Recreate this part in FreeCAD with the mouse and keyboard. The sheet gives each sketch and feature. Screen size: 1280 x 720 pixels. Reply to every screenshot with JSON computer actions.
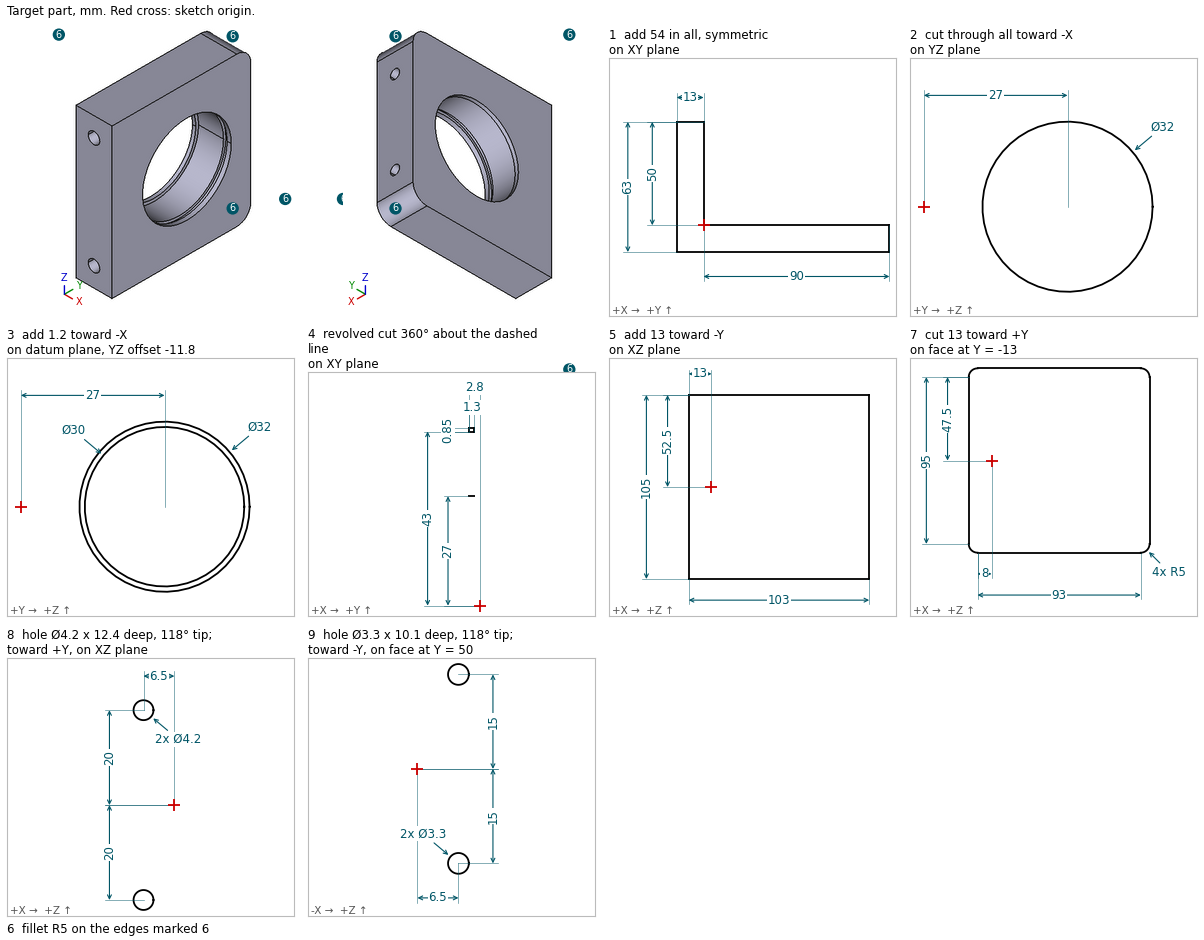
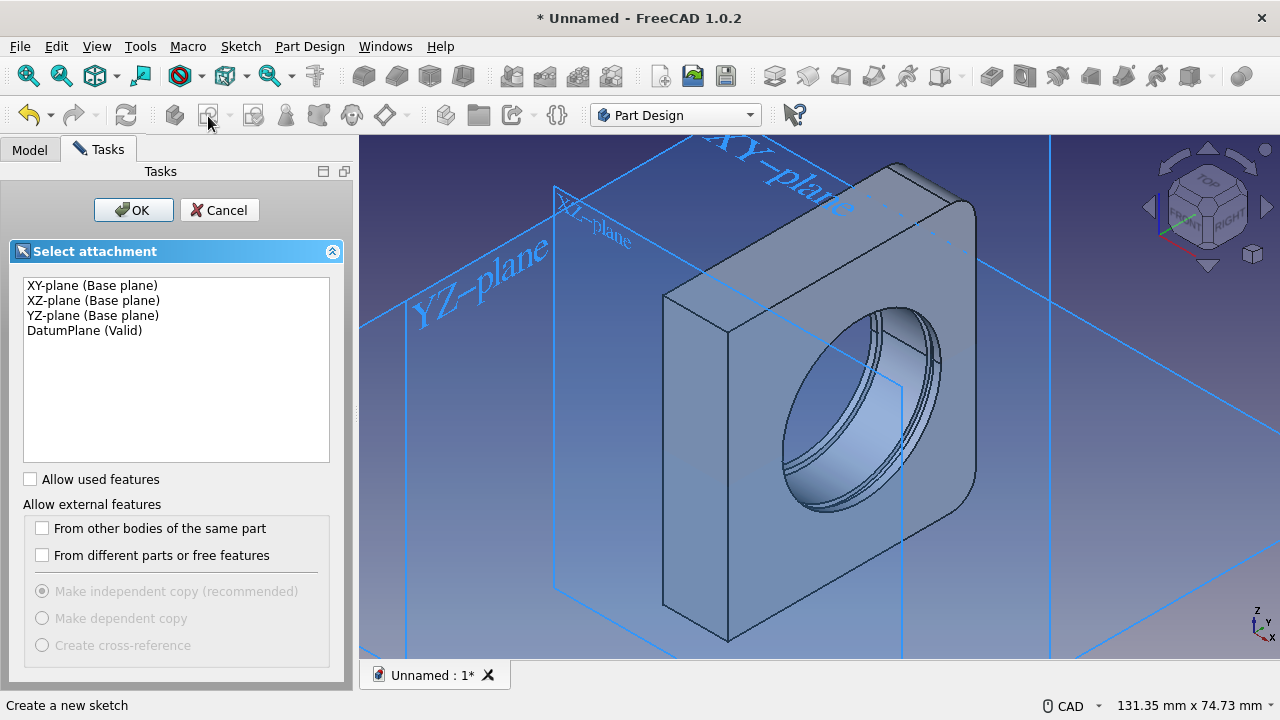
{"action": "left_click", "coordinate": [84, 300]}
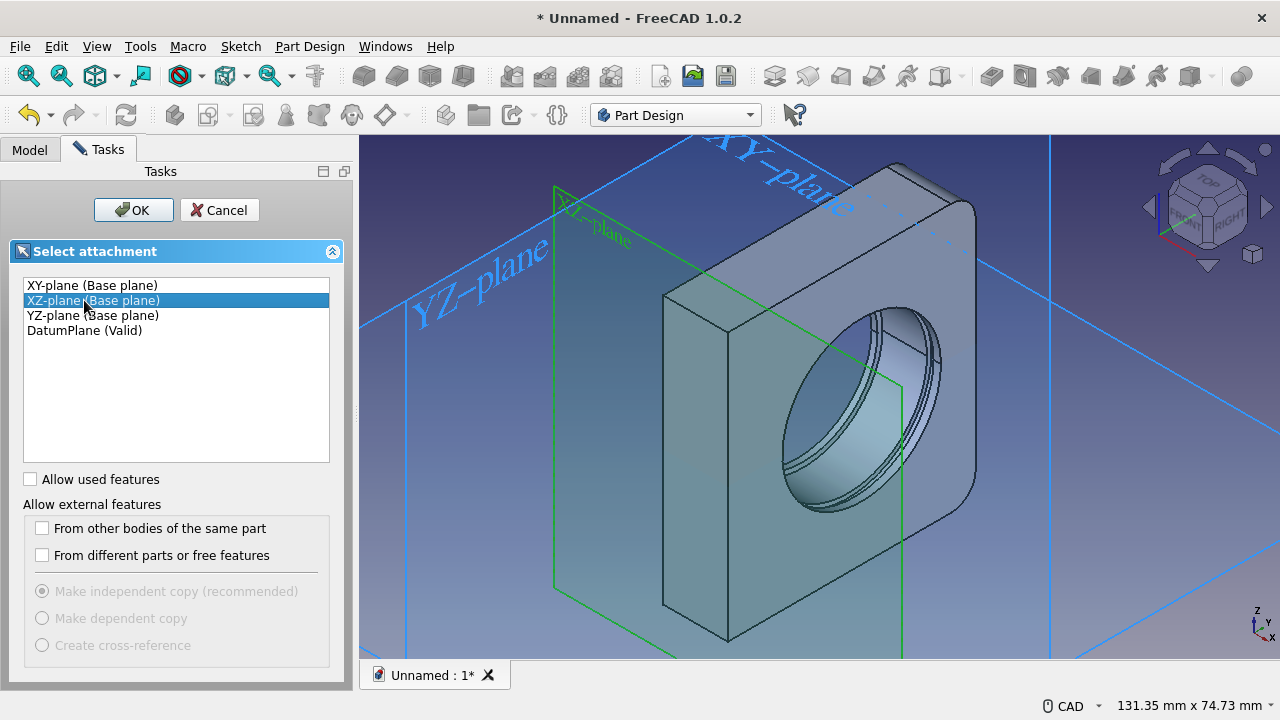
{"action": "left_click", "coordinate": [134, 210]}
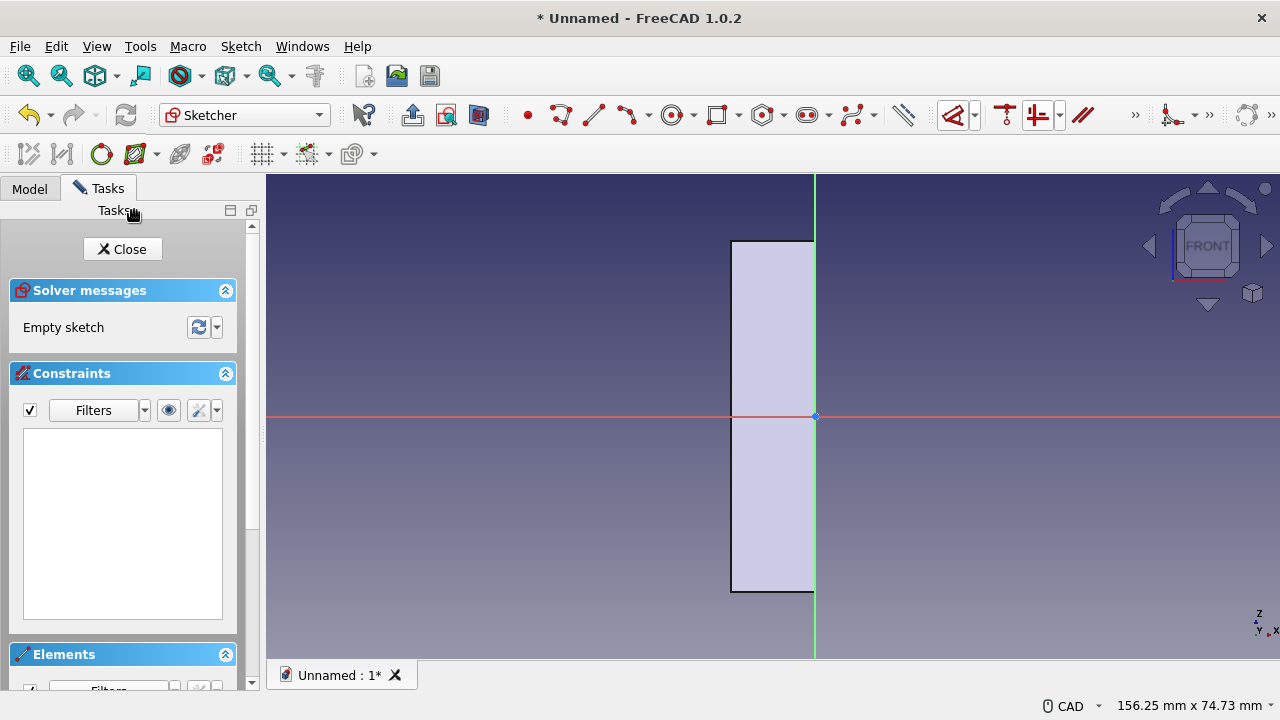
{"action": "left_click", "coordinate": [672, 116]}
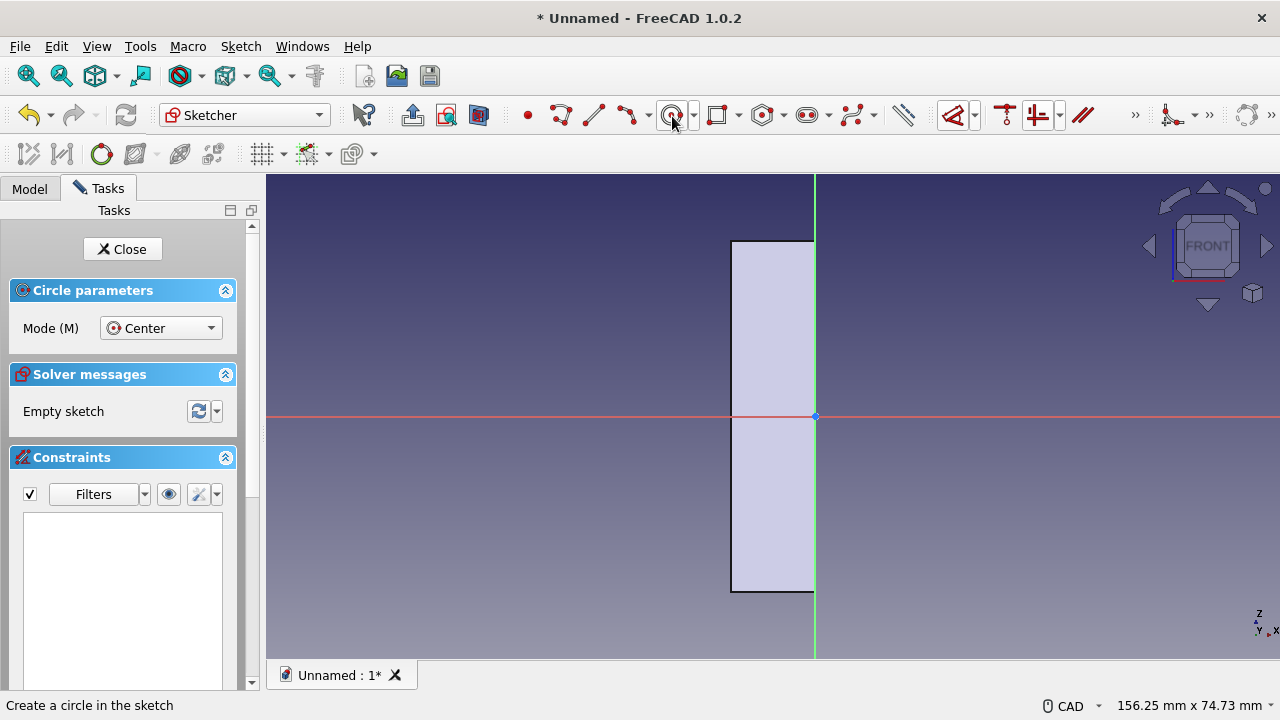
{"action": "scroll", "coordinate": [773, 287], "scroll_direction": "up", "scroll_amount": 3}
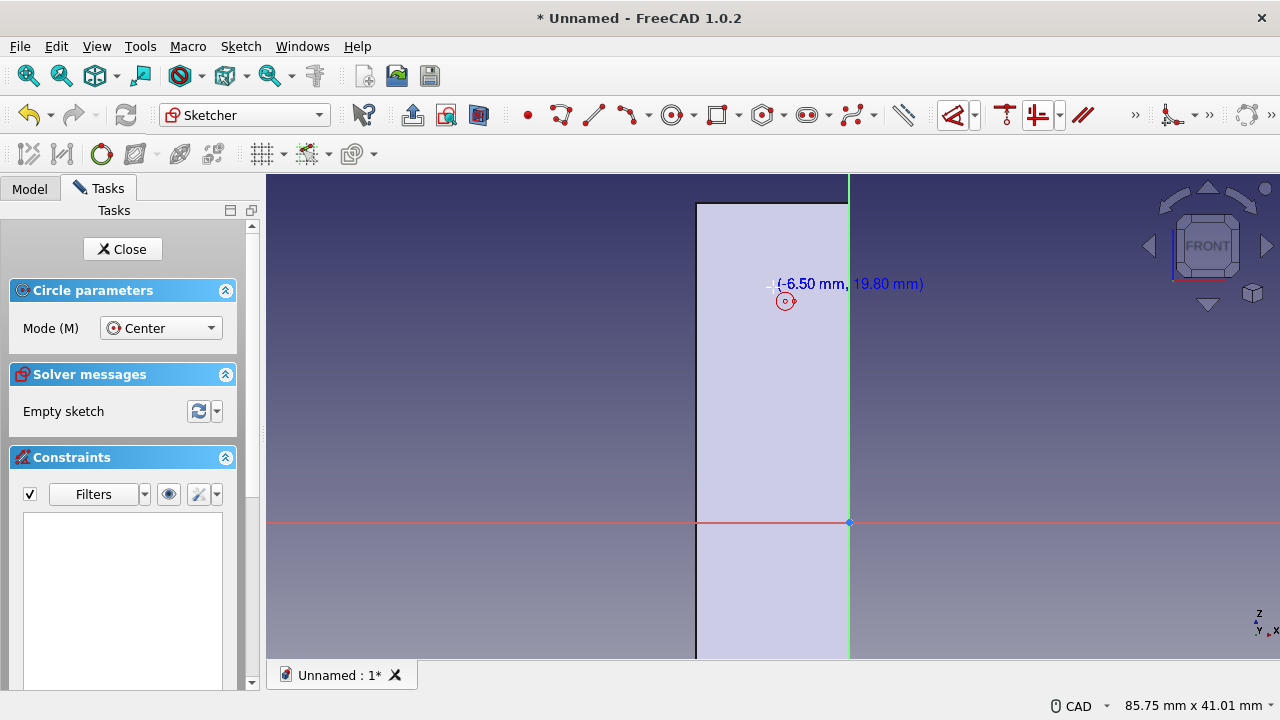
{"action": "left_click", "coordinate": [773, 286]}
{"action": "left_click", "coordinate": [790, 269]}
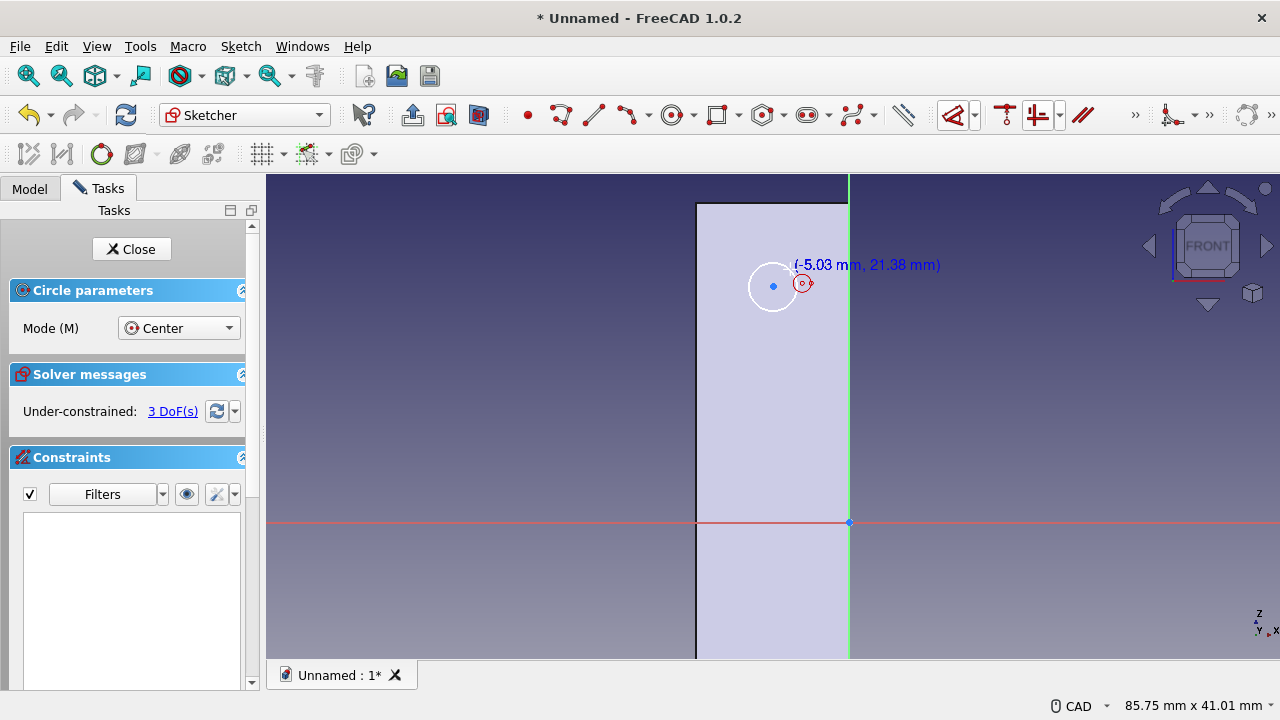
{"action": "scroll", "coordinate": [590, 287], "scroll_direction": "down", "scroll_amount": 3}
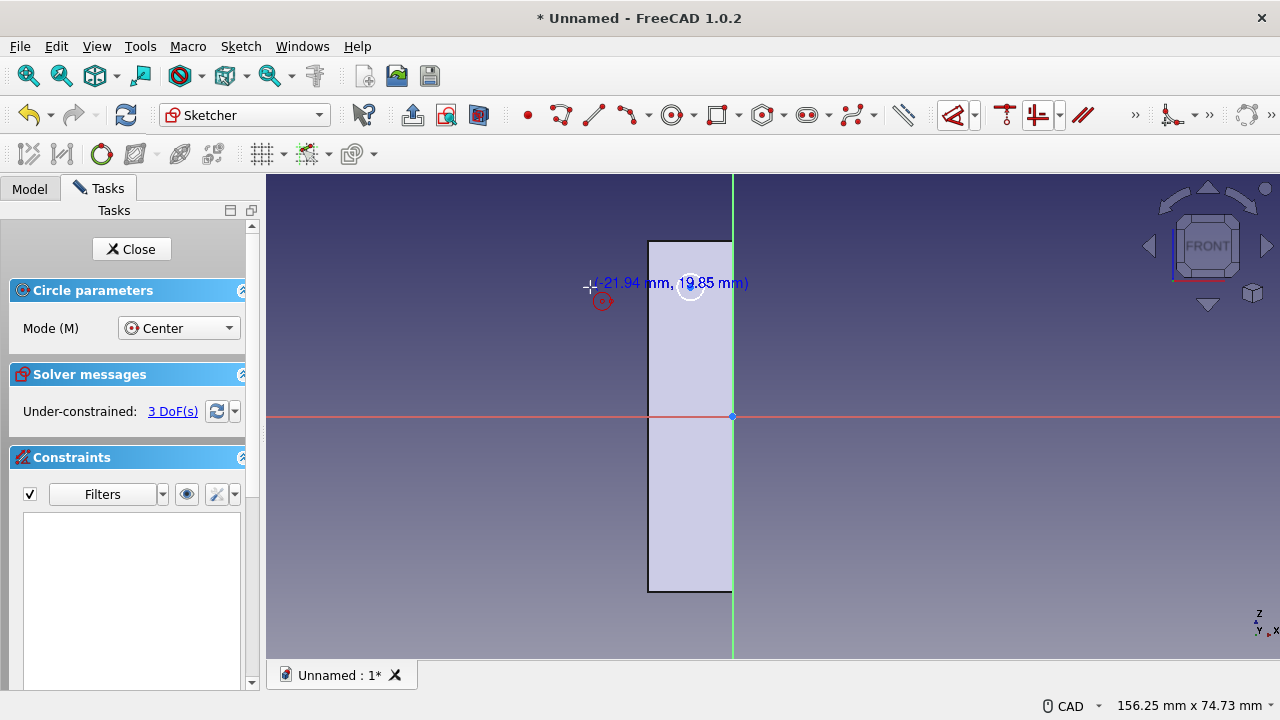
{"action": "scroll", "coordinate": [690, 546], "scroll_direction": "up", "scroll_amount": 3}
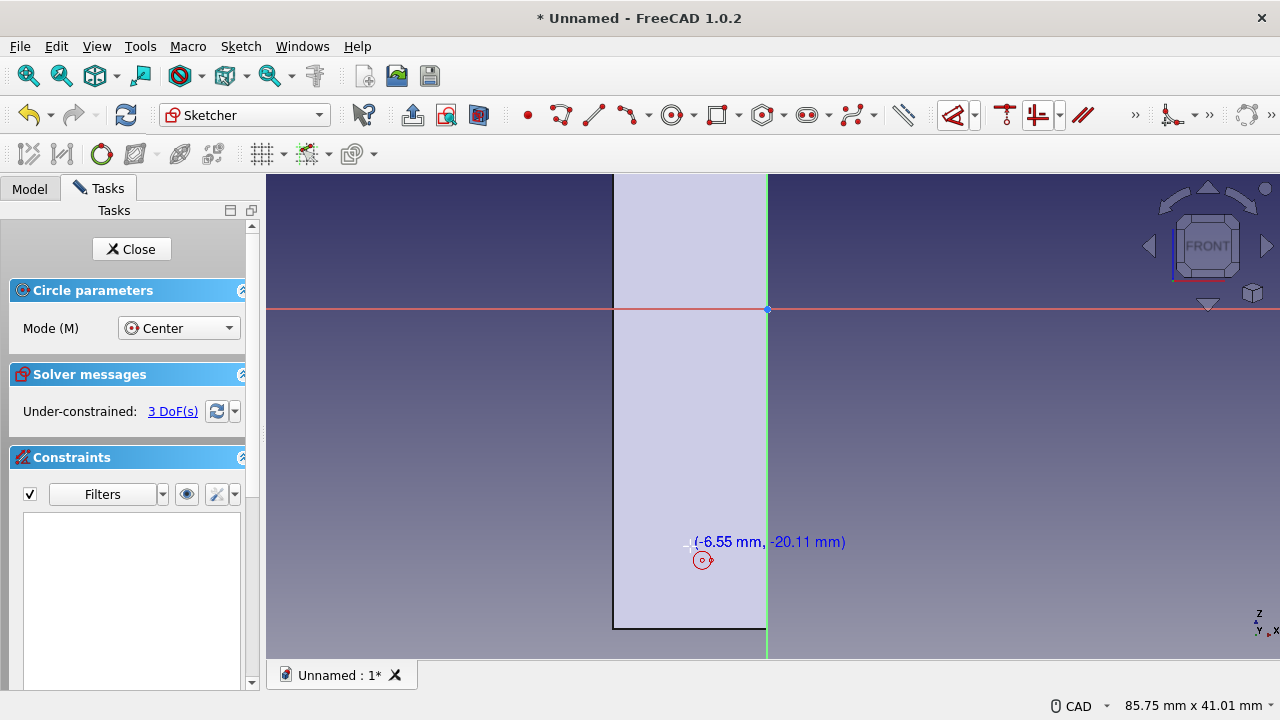
{"action": "left_click", "coordinate": [690, 546]}
{"action": "left_click", "coordinate": [708, 528]}
{"action": "key", "text": "Escape"}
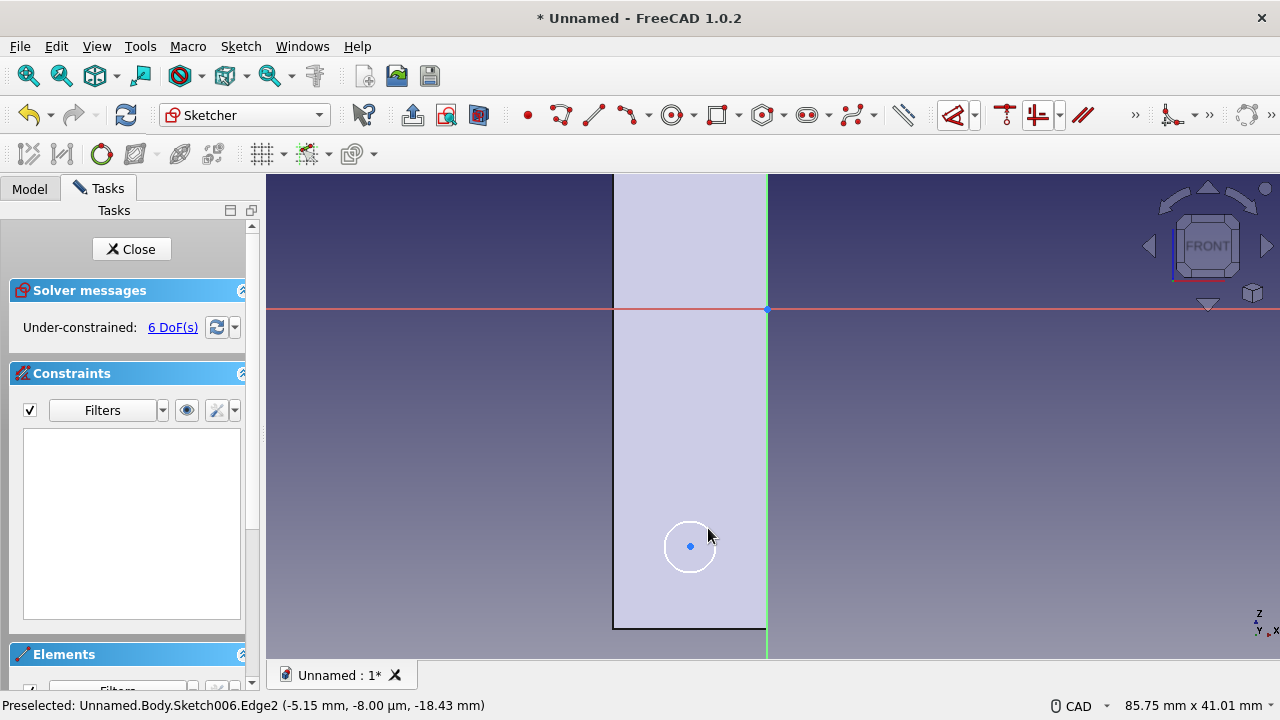
{"action": "scroll", "coordinate": [690, 547], "scroll_direction": "down", "scroll_amount": 3}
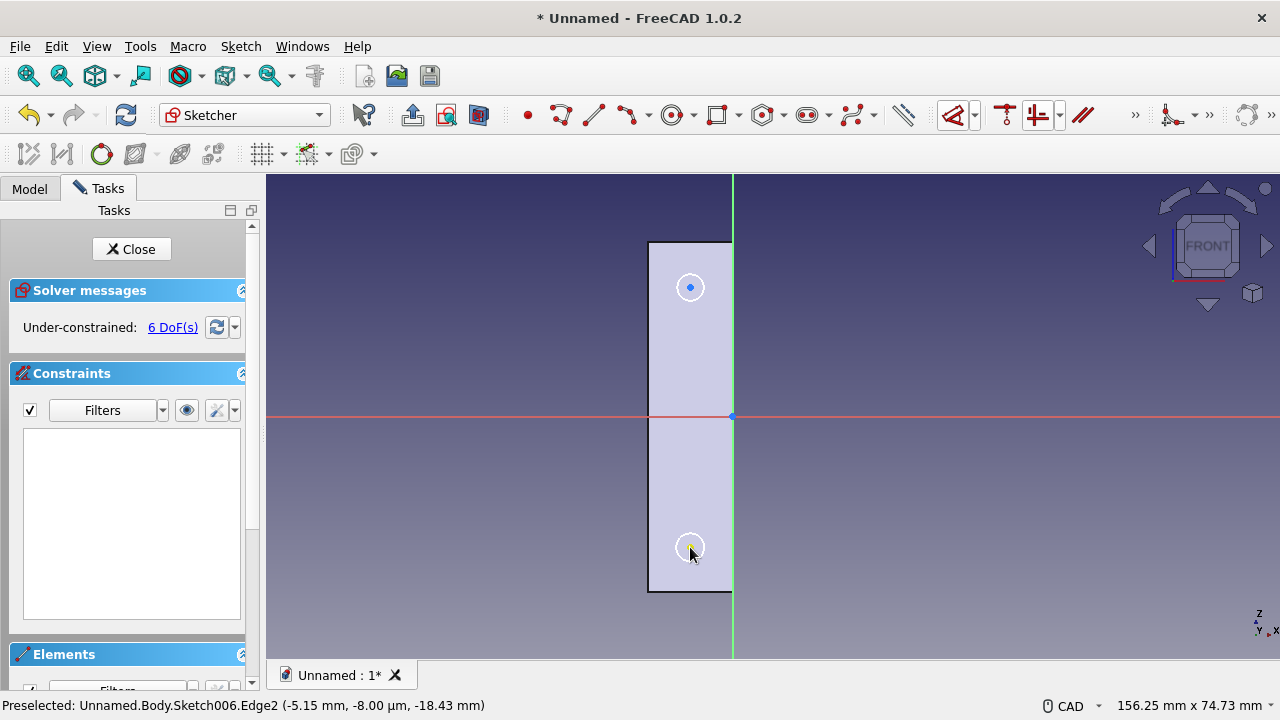
{"action": "left_click", "coordinate": [700, 278]}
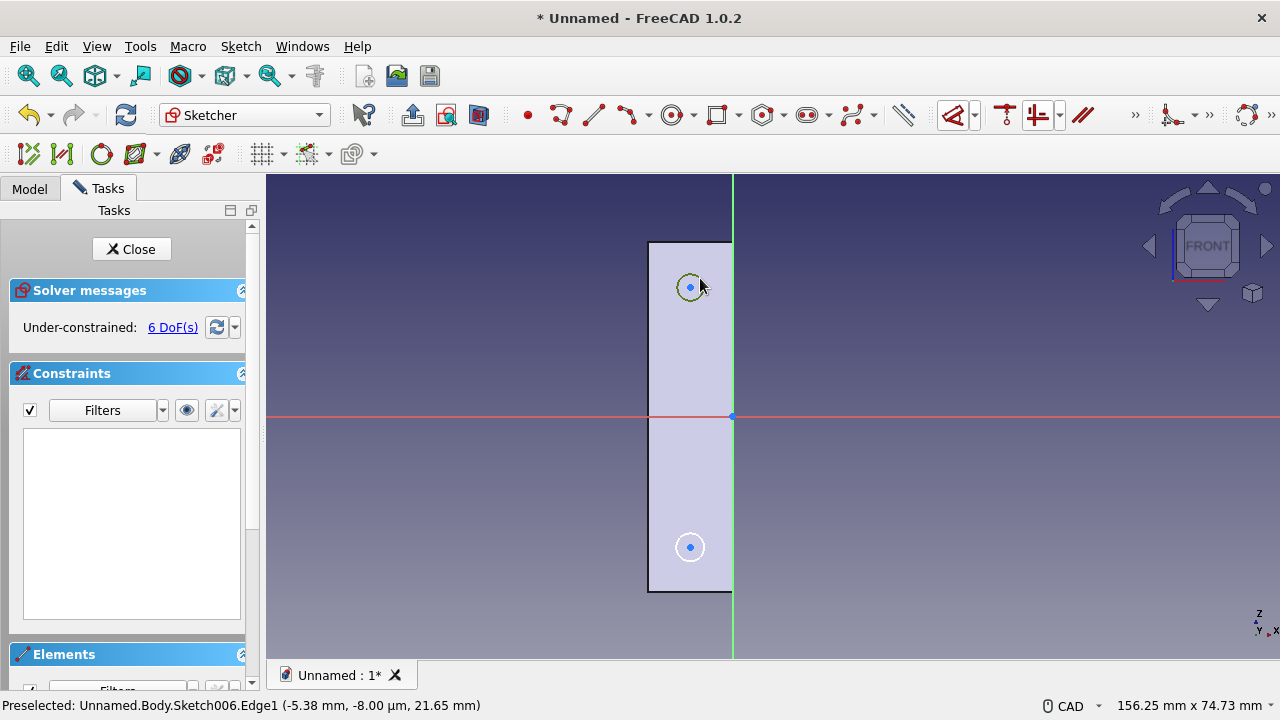
{"action": "left_click", "coordinate": [700, 537]}